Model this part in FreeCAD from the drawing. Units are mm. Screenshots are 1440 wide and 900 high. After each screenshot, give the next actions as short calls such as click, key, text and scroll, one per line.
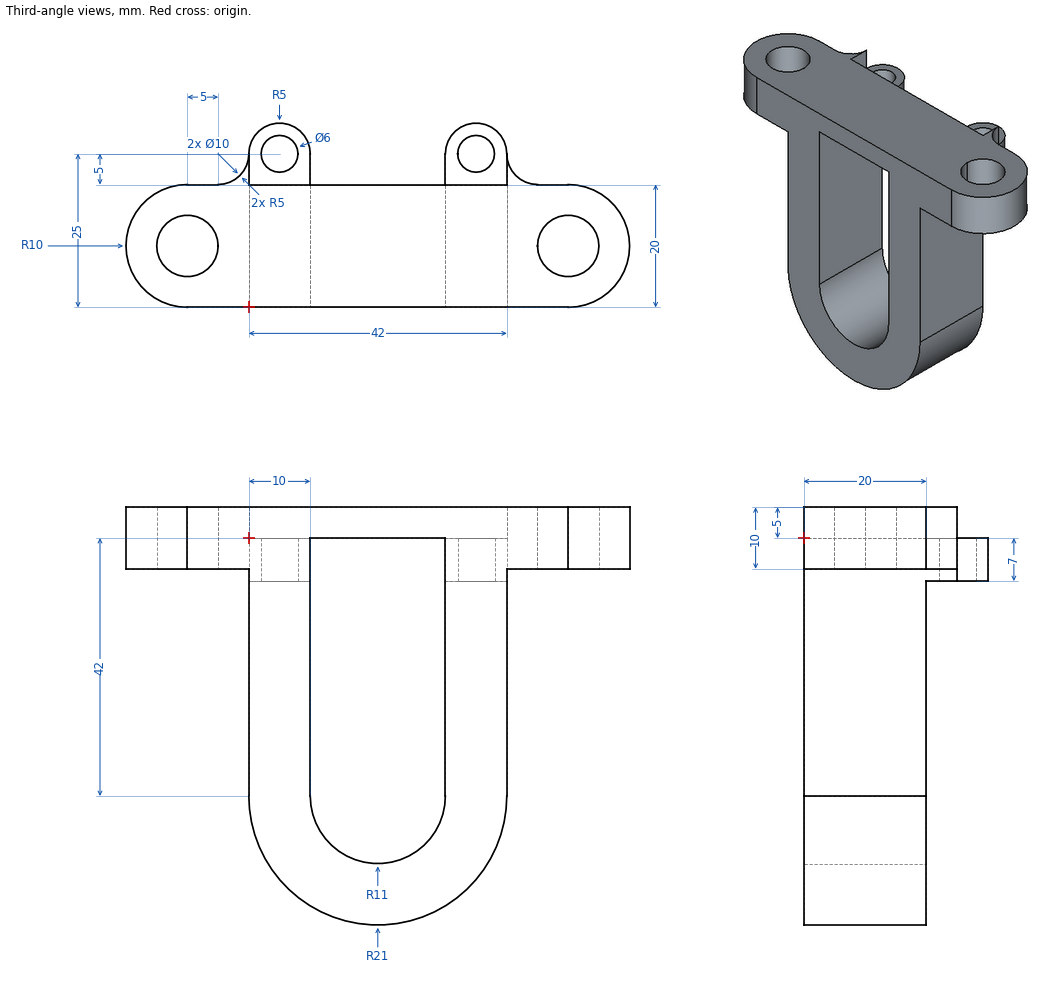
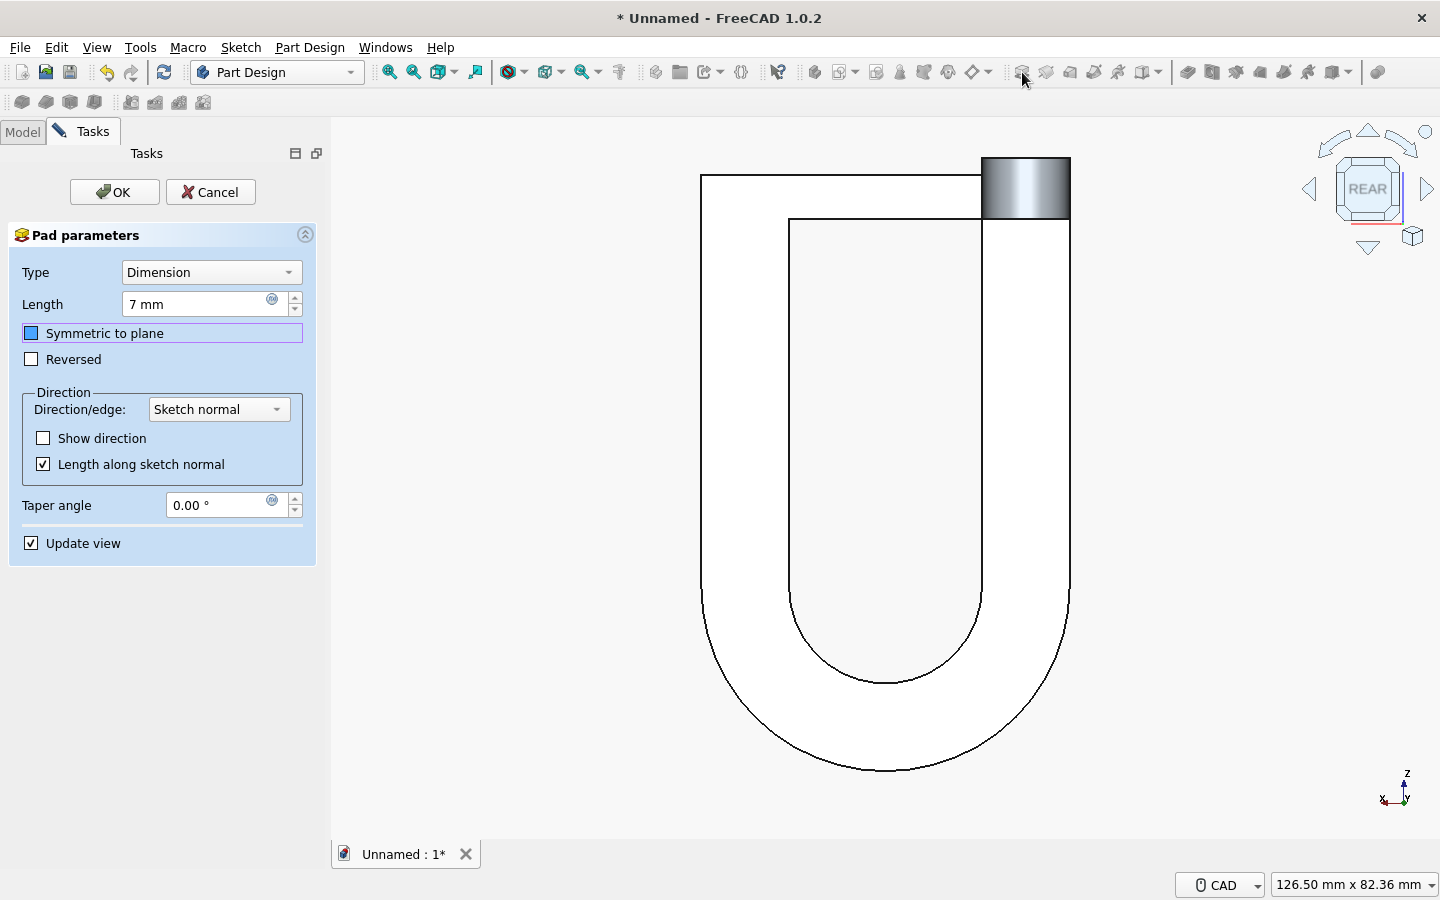
click(30, 359)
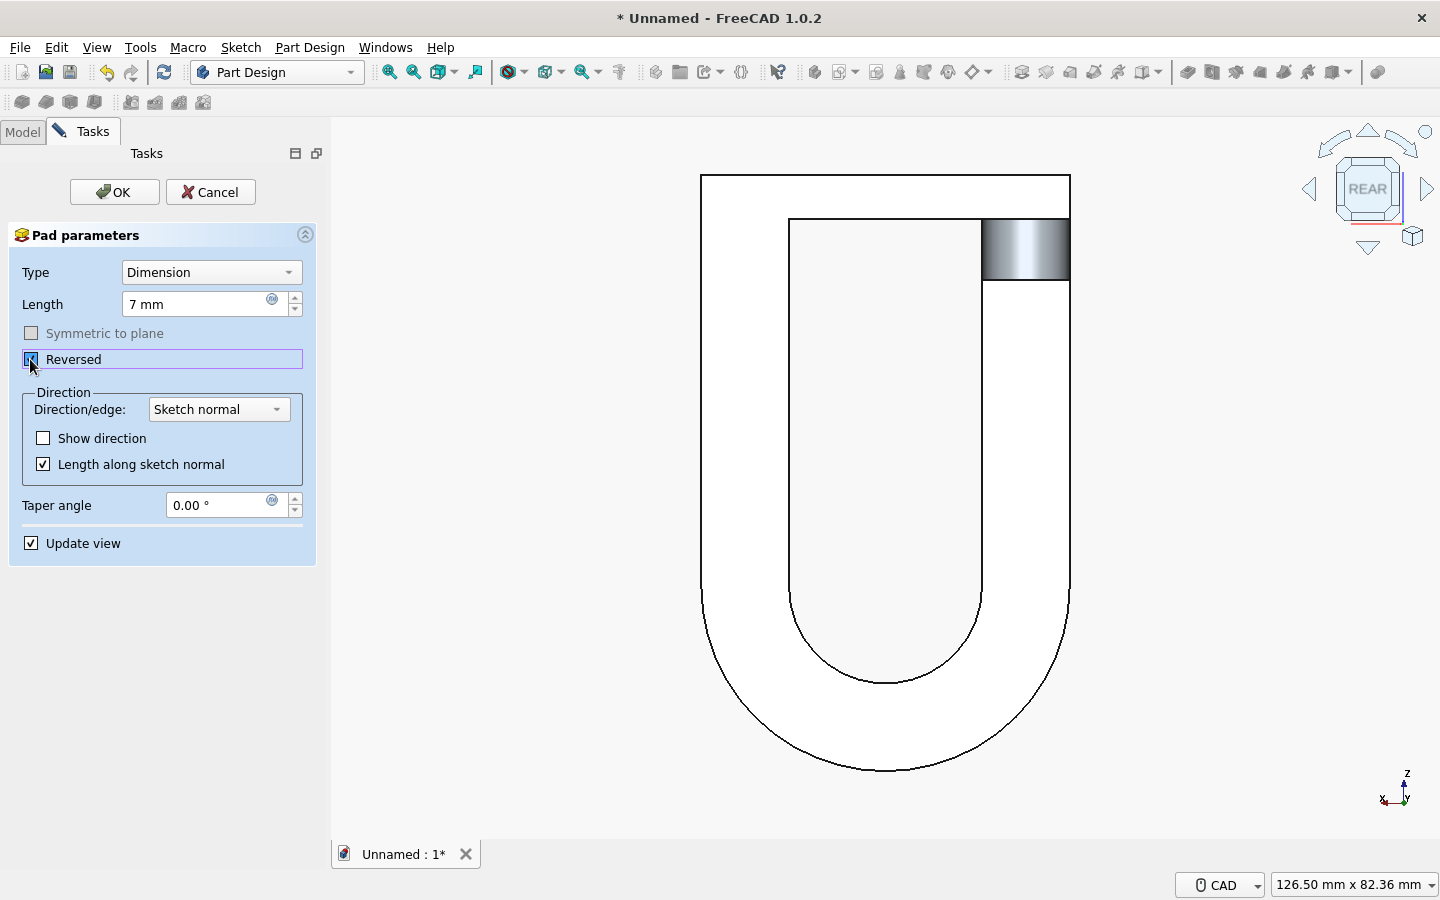
click(115, 192)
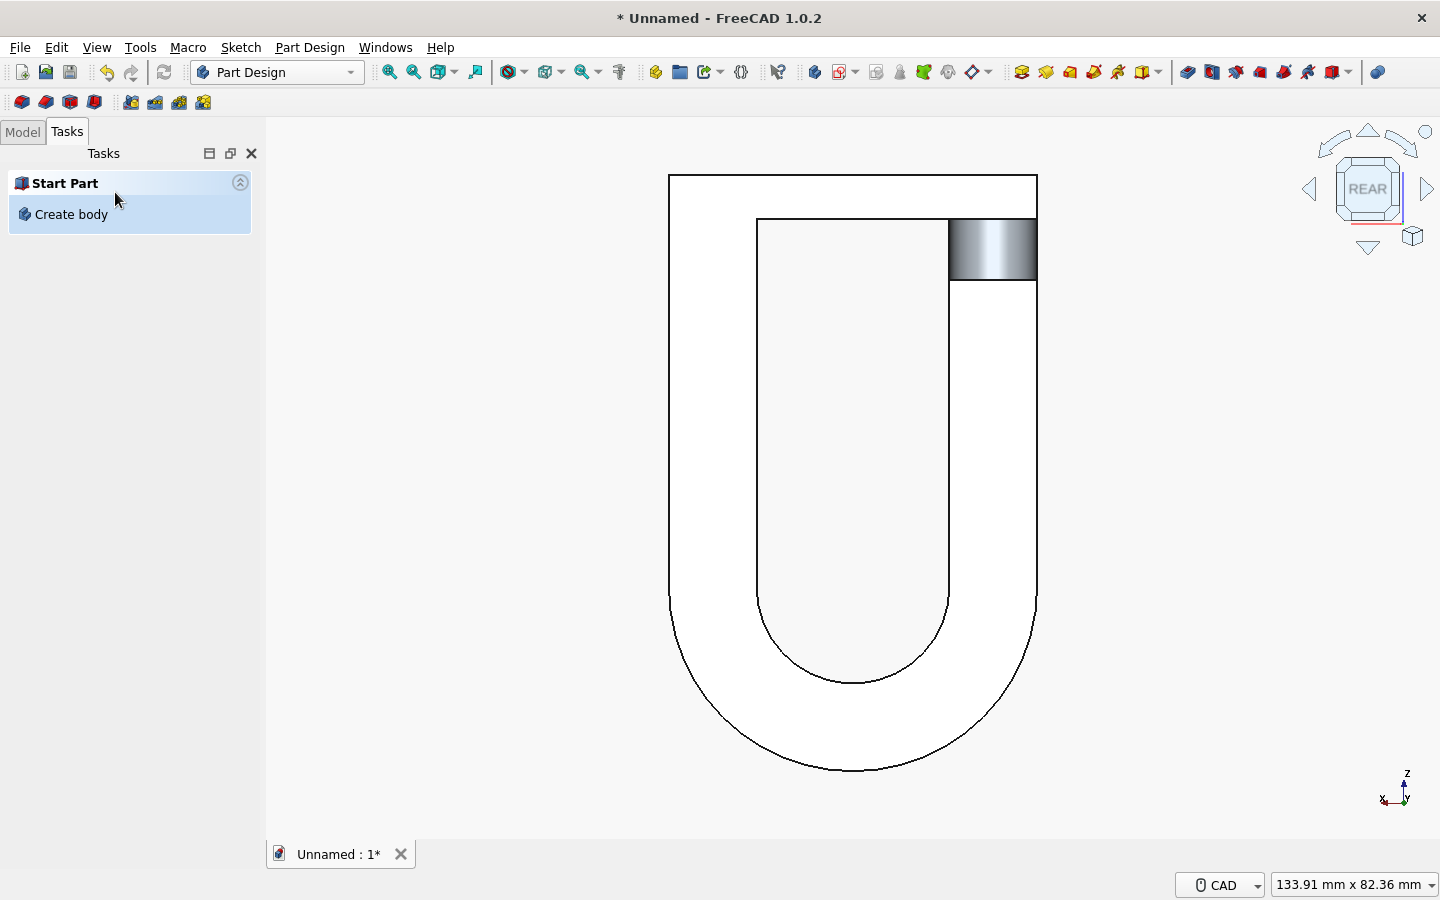
click(23, 131)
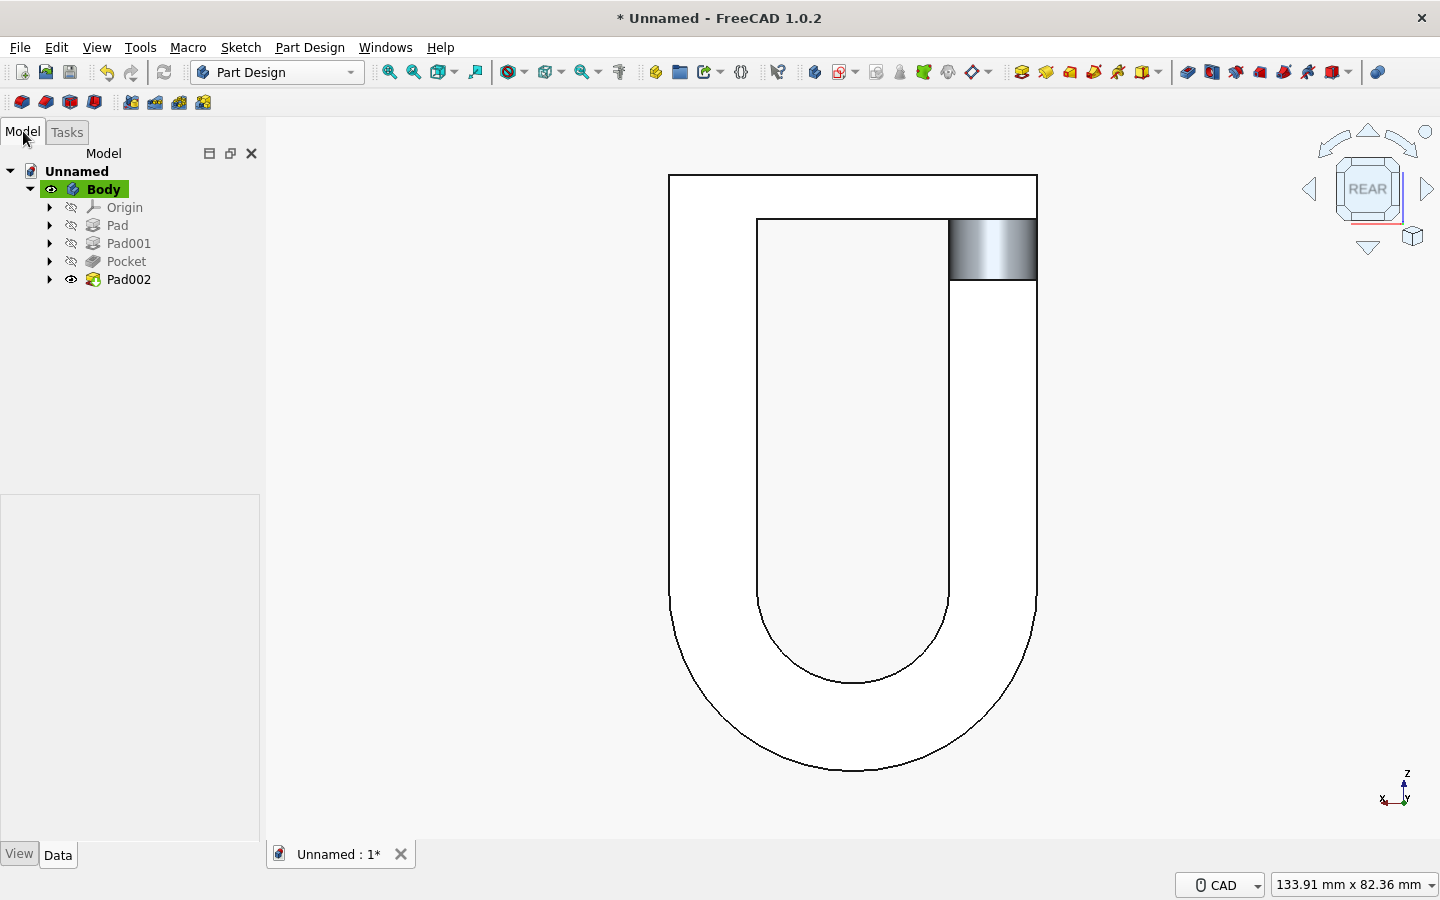
click(50, 207)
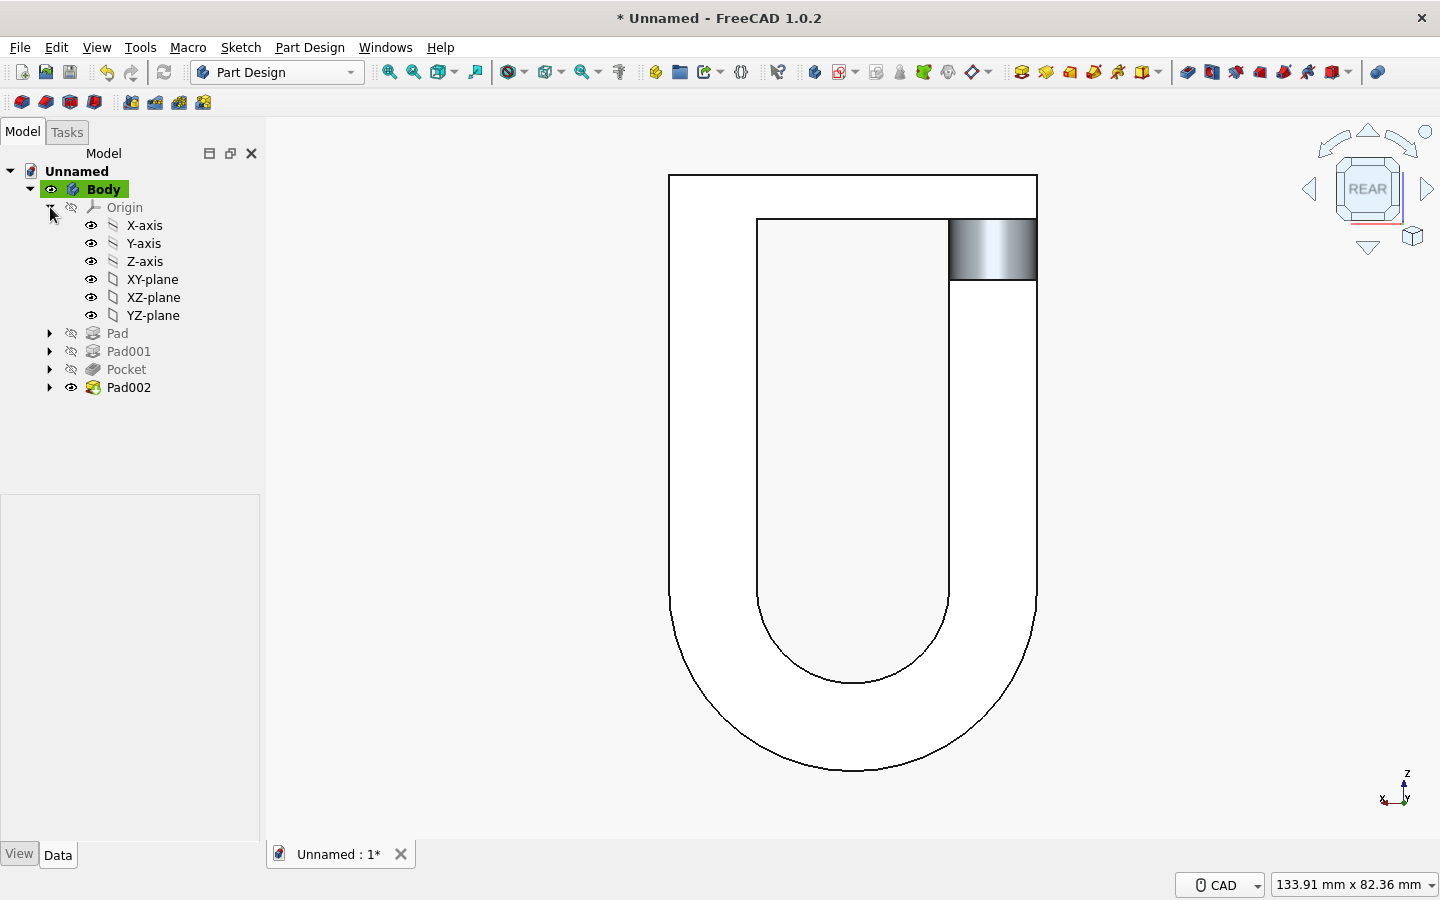
click(136, 315)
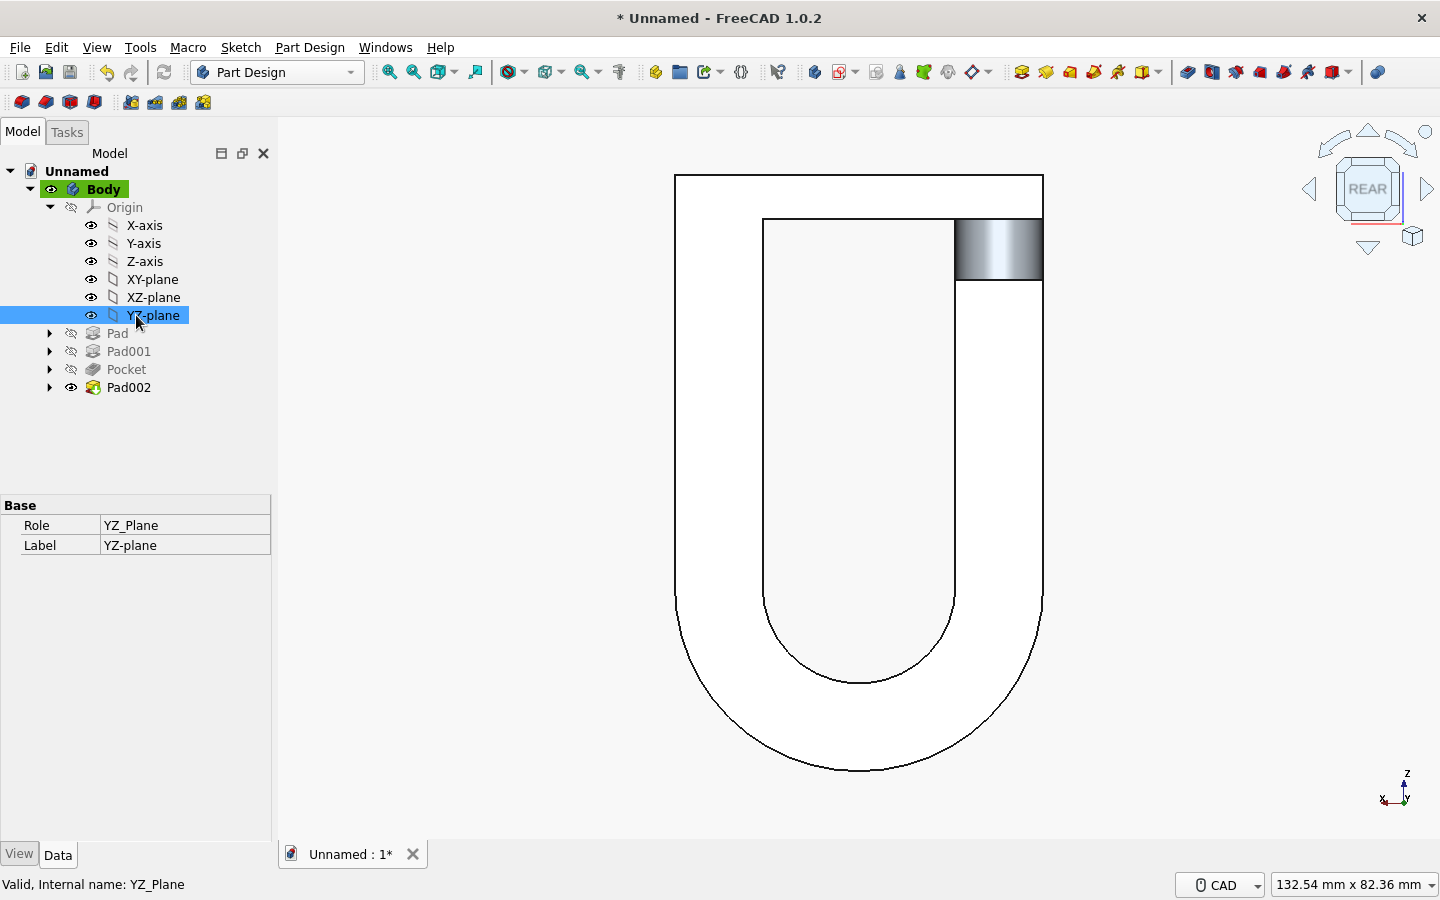
click(972, 72)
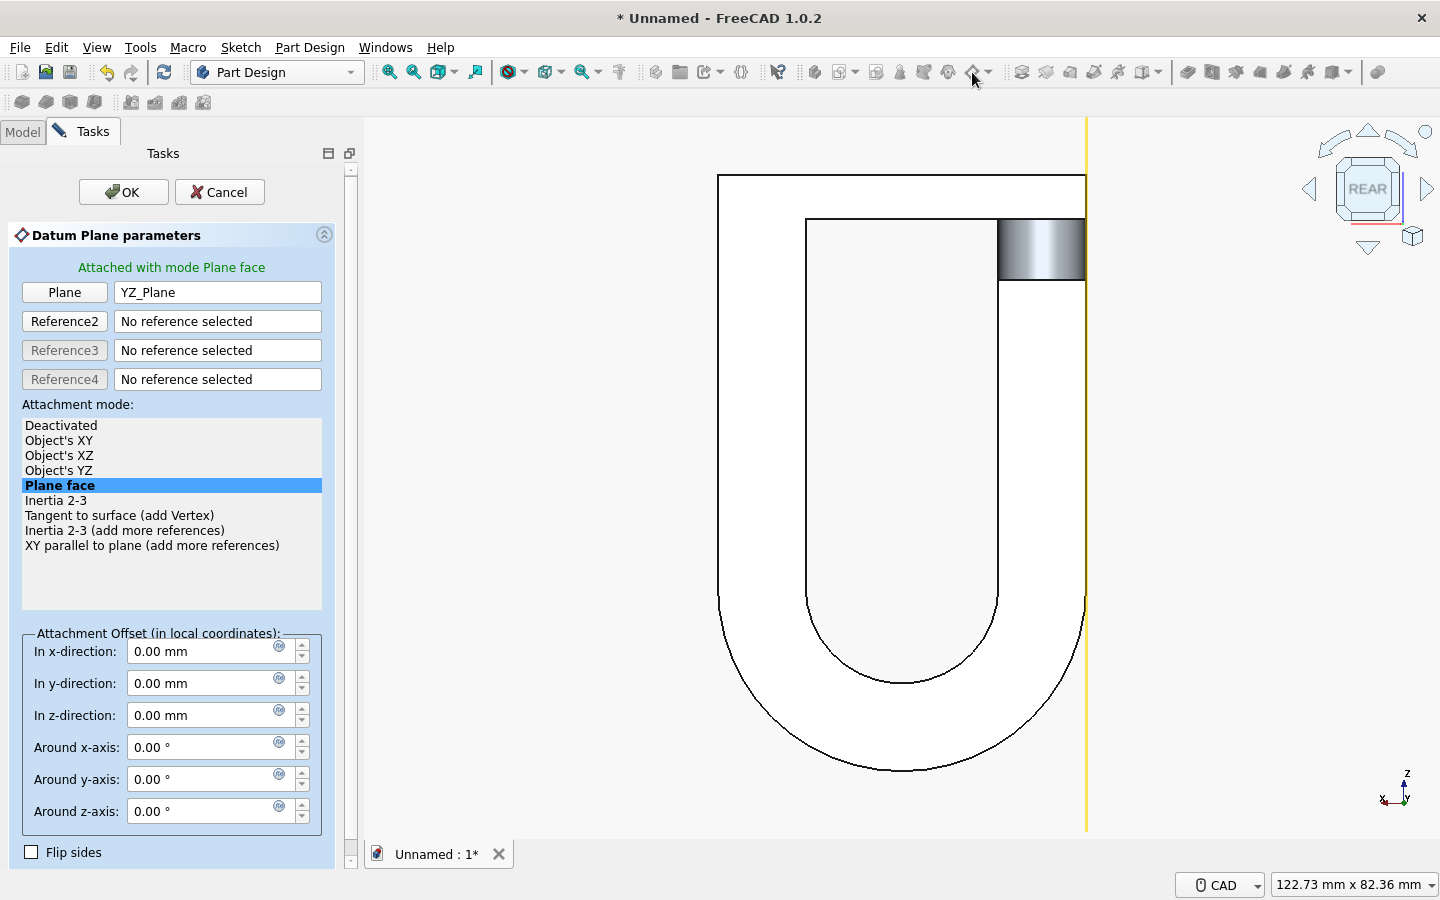
triple_click(210, 715)